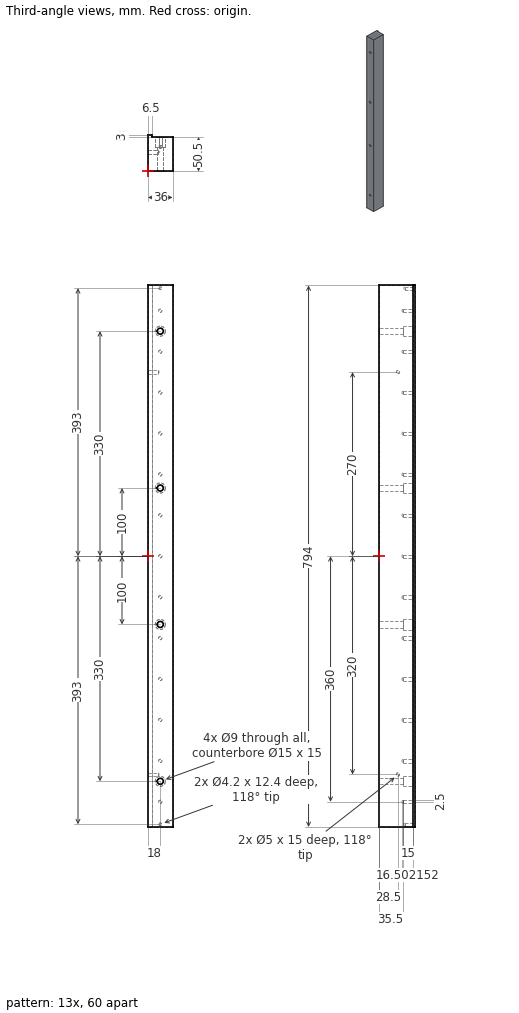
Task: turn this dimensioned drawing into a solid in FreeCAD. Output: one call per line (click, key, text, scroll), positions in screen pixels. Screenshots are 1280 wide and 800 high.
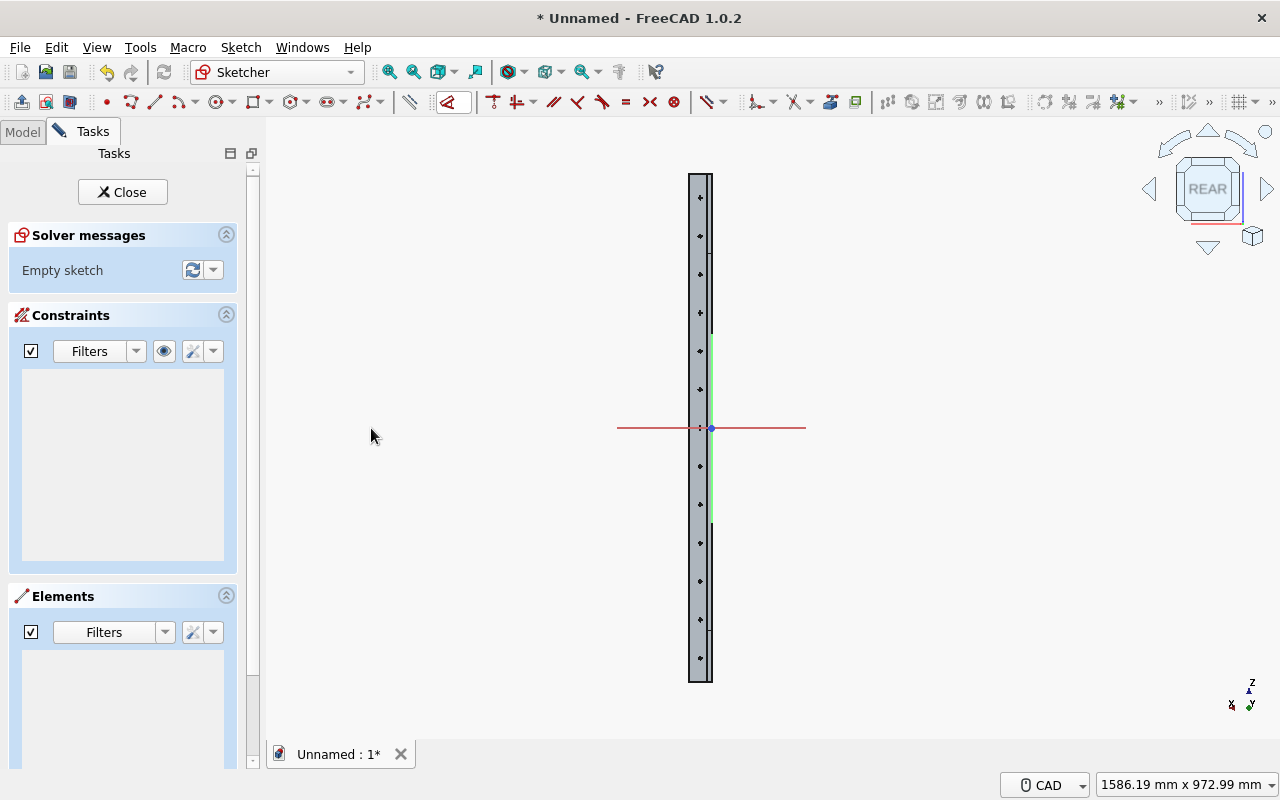
click(216, 102)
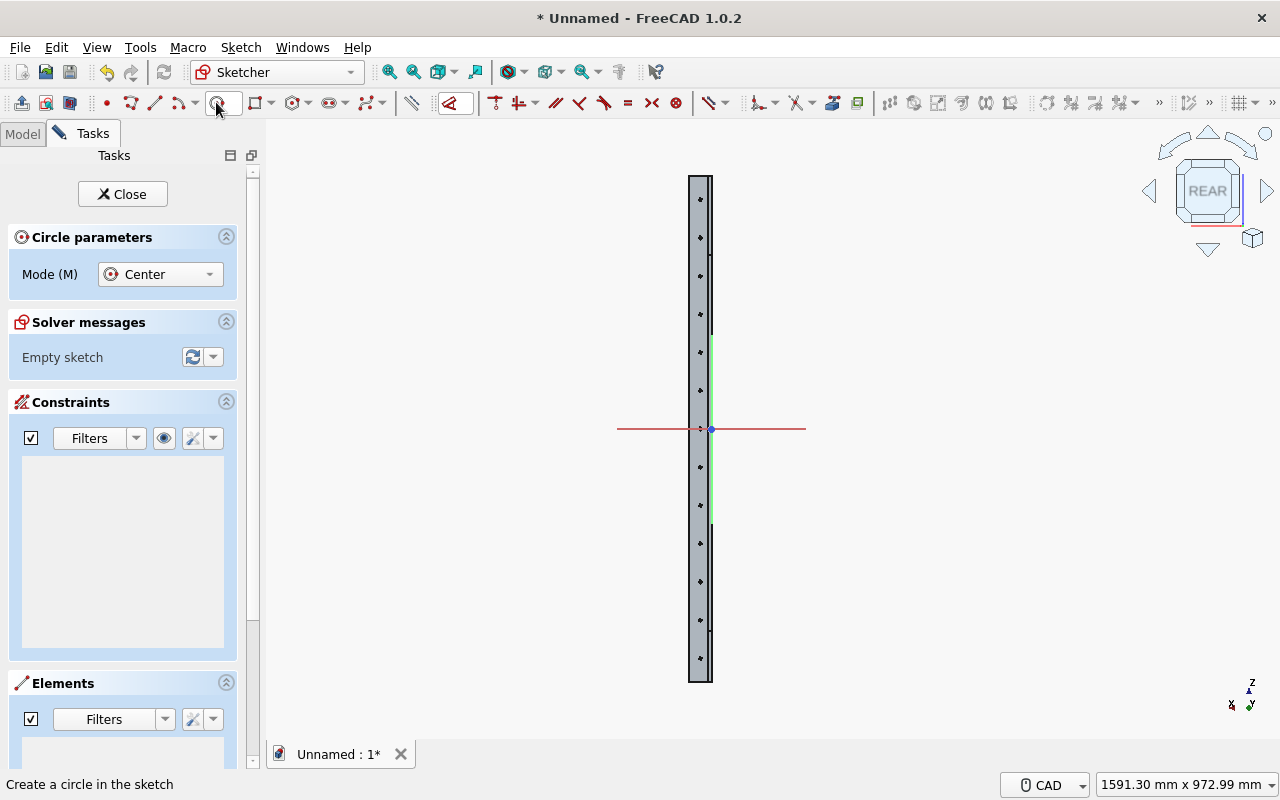
scroll(700, 639, up, 11)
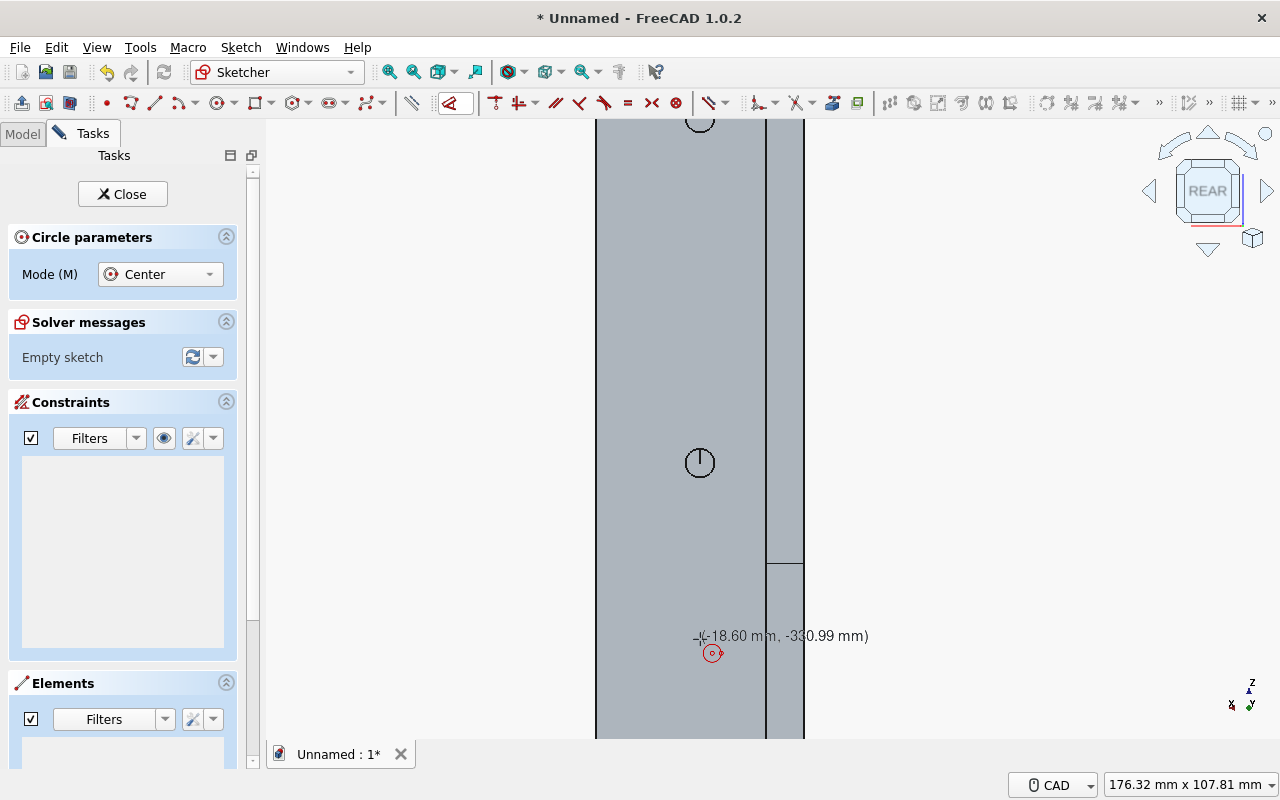
scroll(700, 640, down, 11)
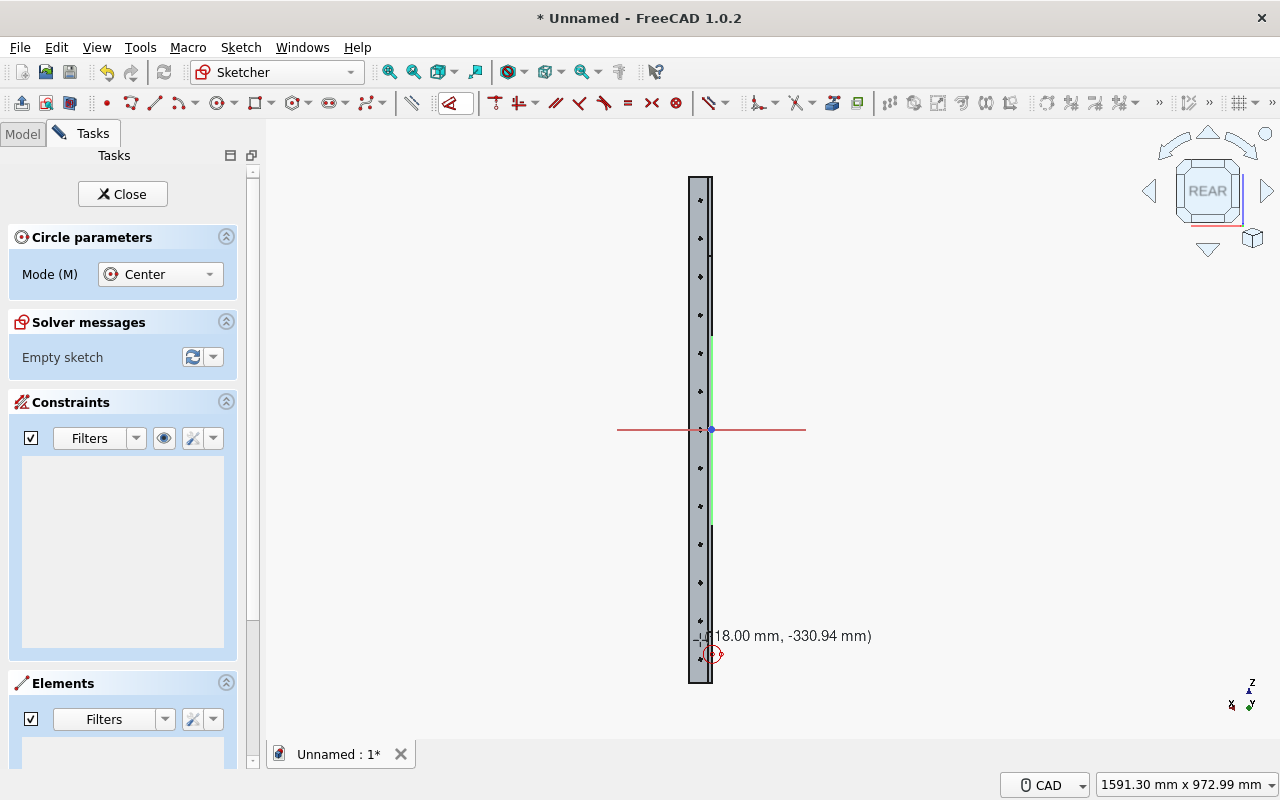
scroll(700, 640, up, 2)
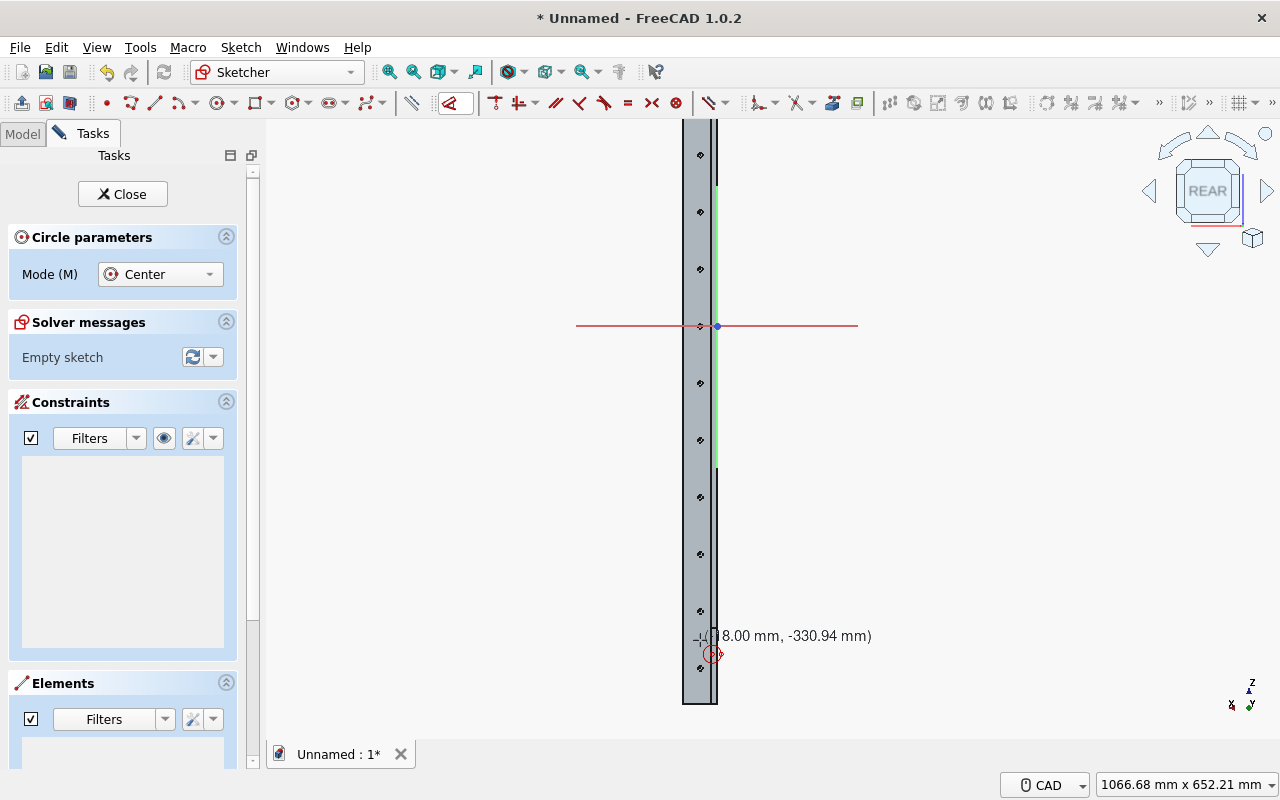
click(700, 640)
move(703, 637)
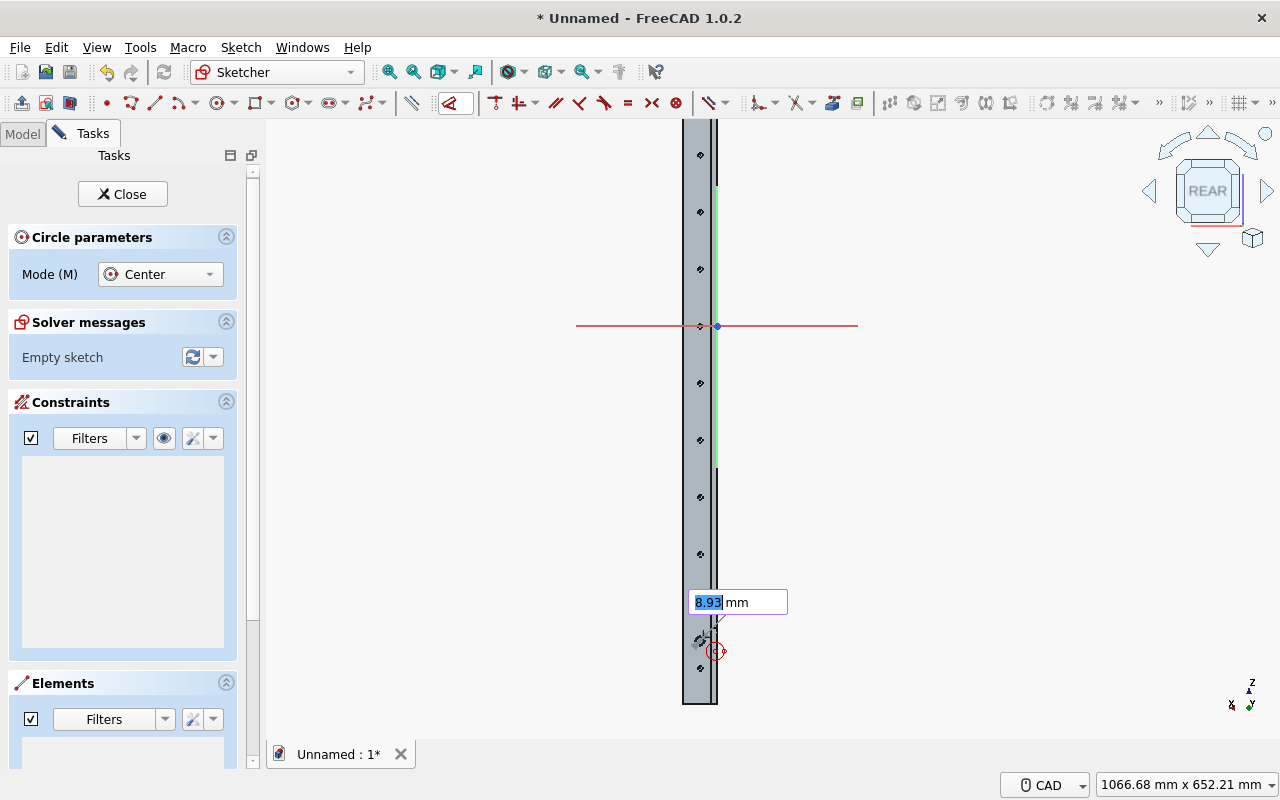
text(9)
key(Return)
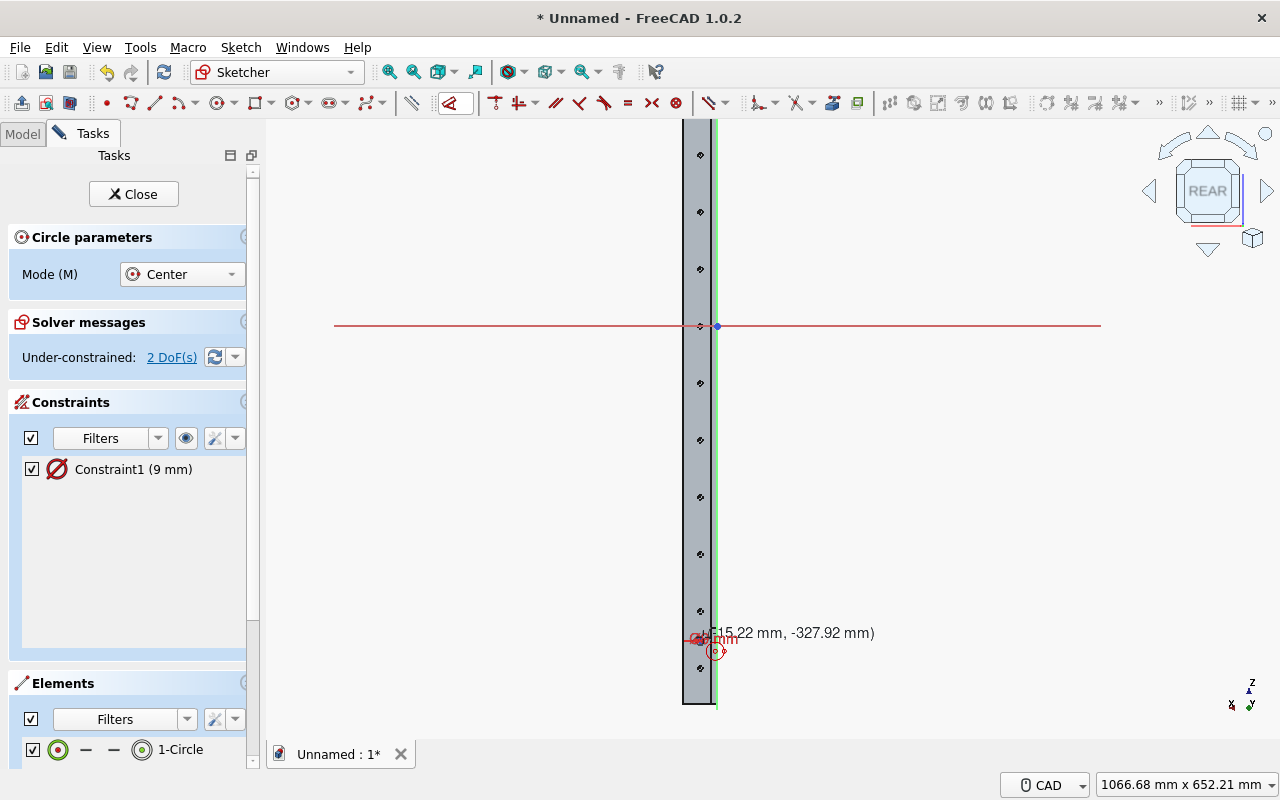
scroll(700, 421, up, 9)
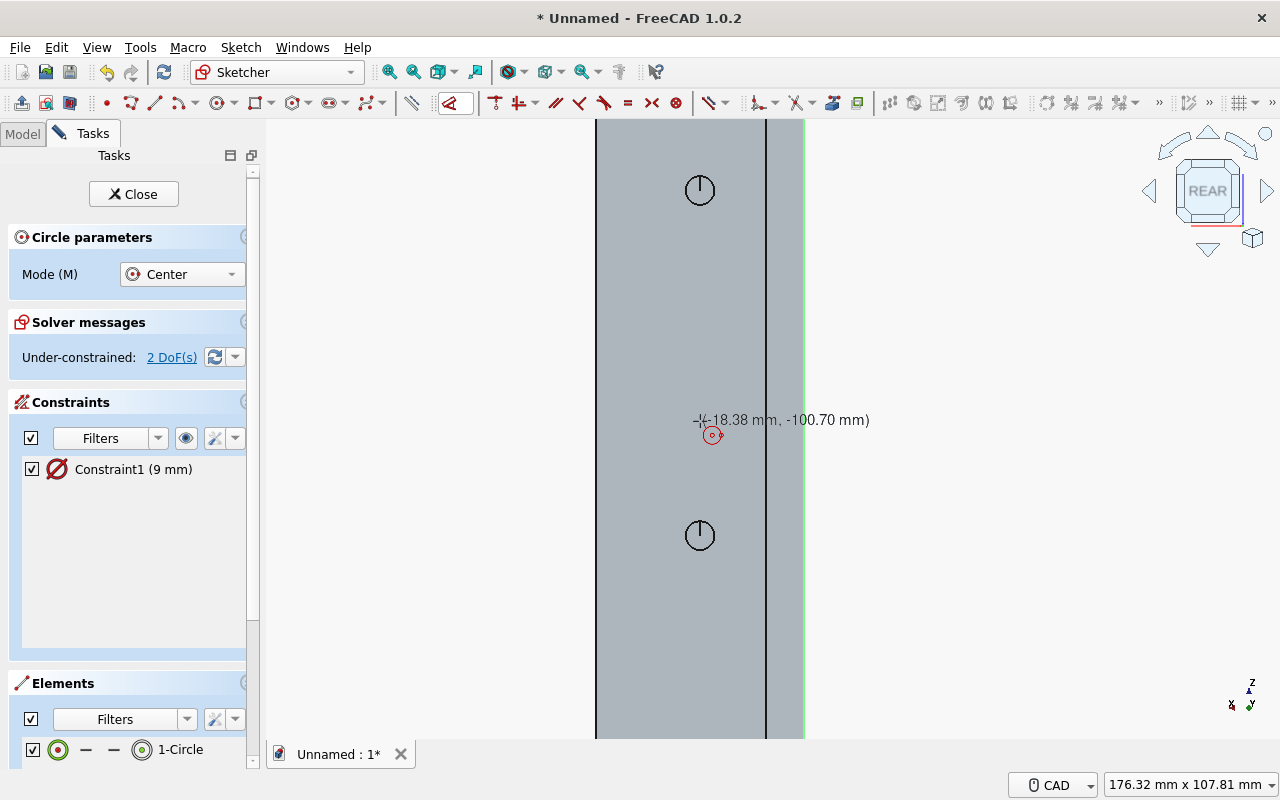
scroll(700, 502, down, 11)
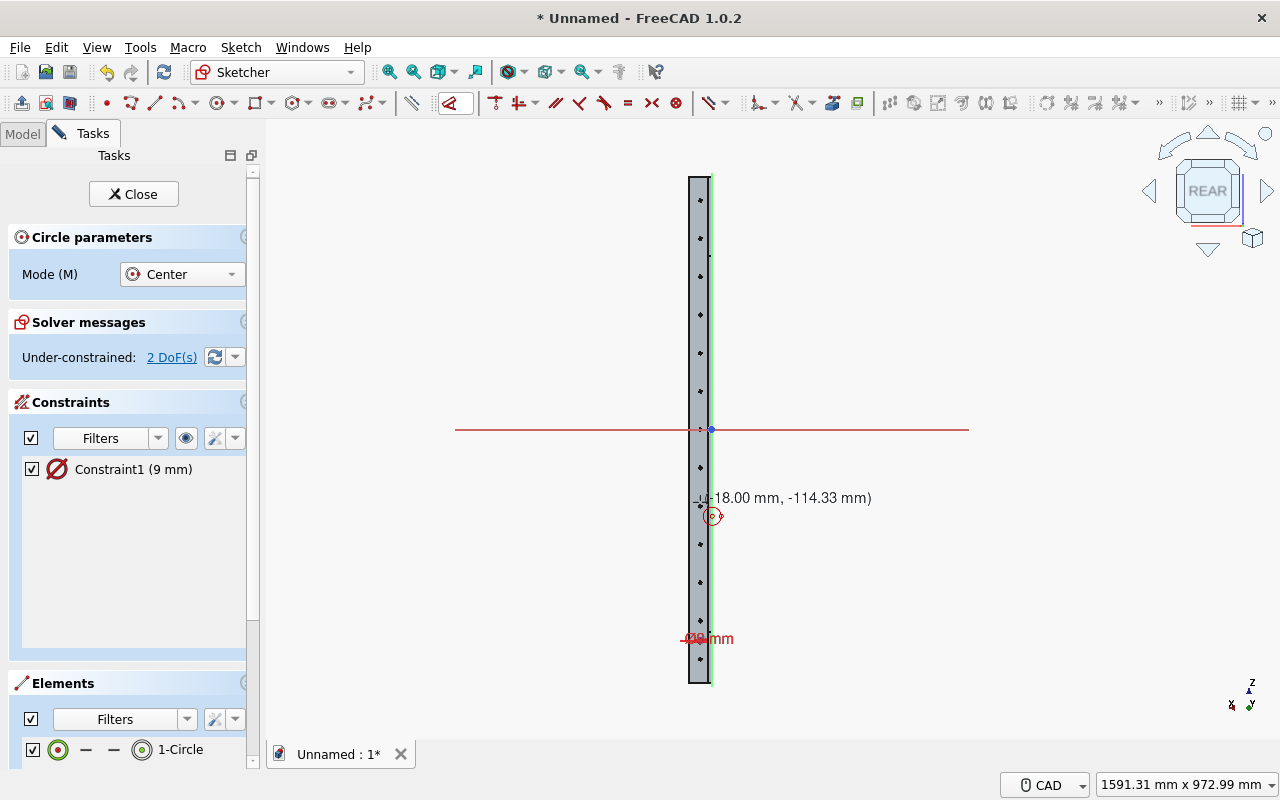
scroll(700, 494, up, 2)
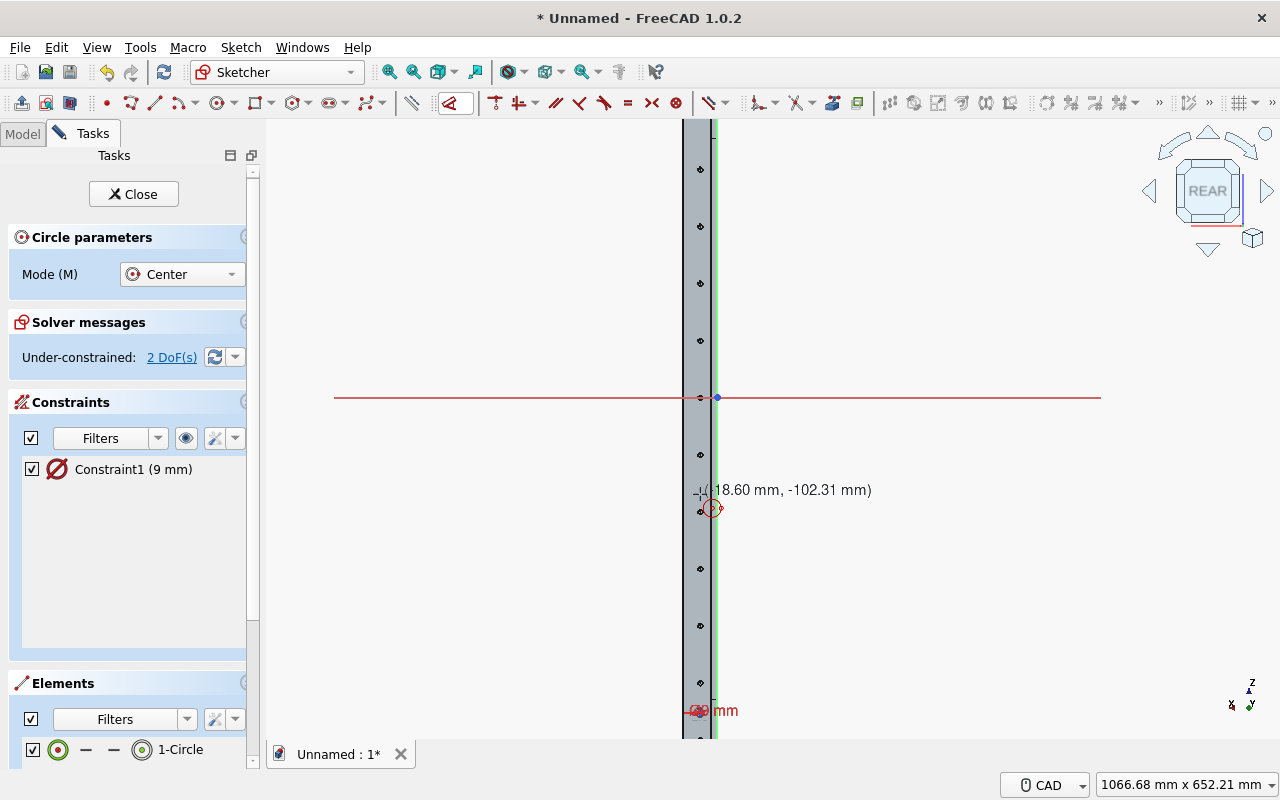
click(700, 493)
move(703, 490)